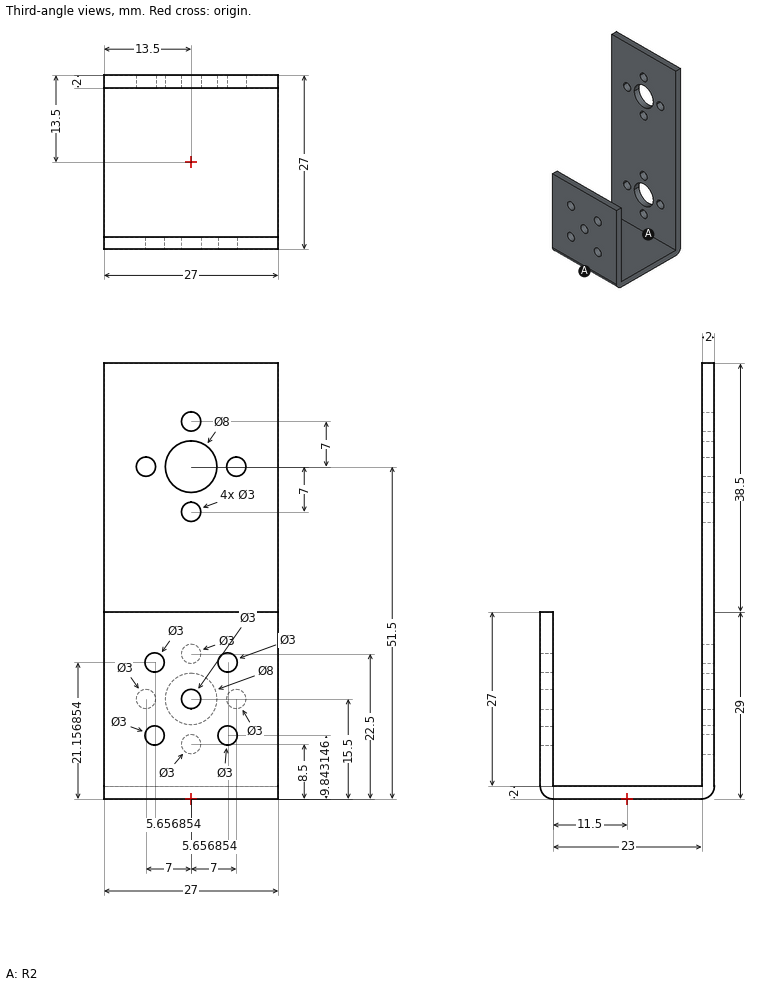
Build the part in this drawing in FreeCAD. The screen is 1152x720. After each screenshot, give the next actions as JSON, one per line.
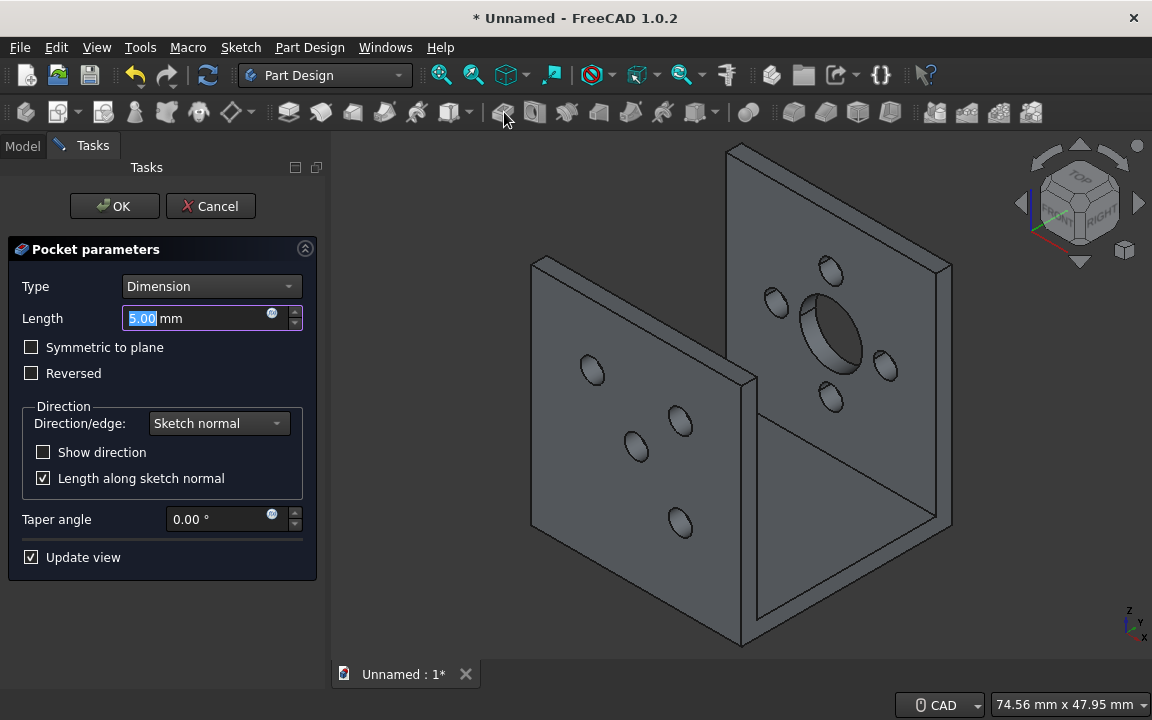
{"action": "left_click", "coordinate": [212, 286]}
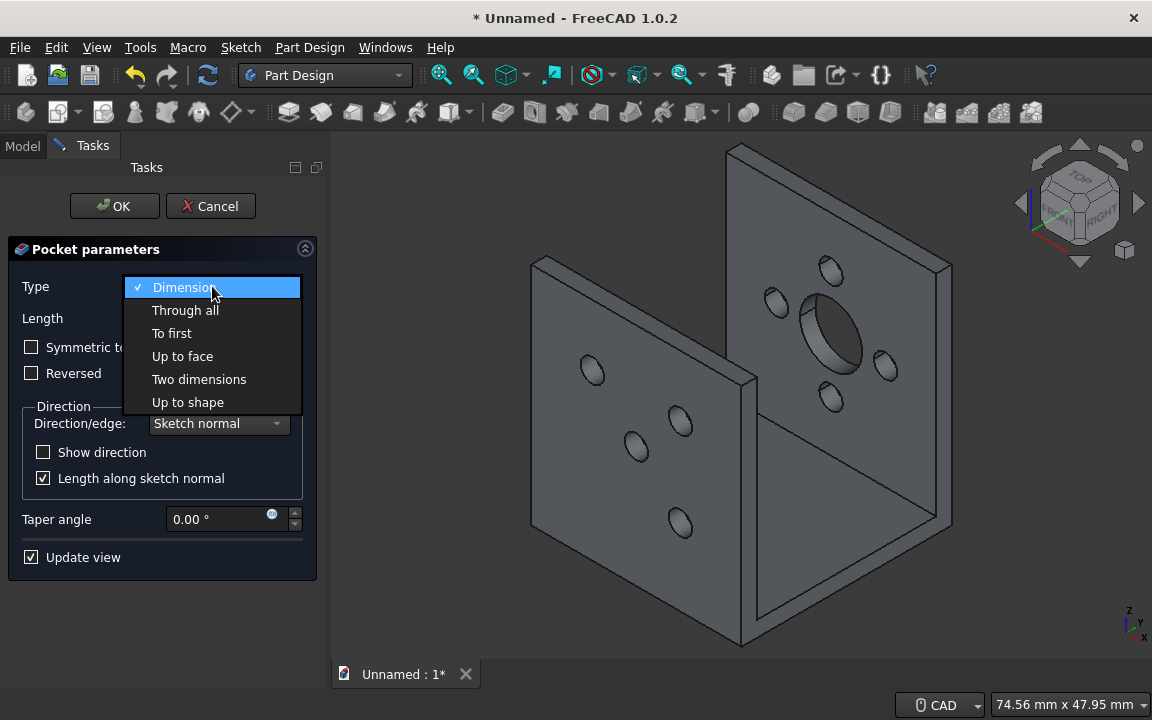
{"action": "left_click", "coordinate": [212, 334]}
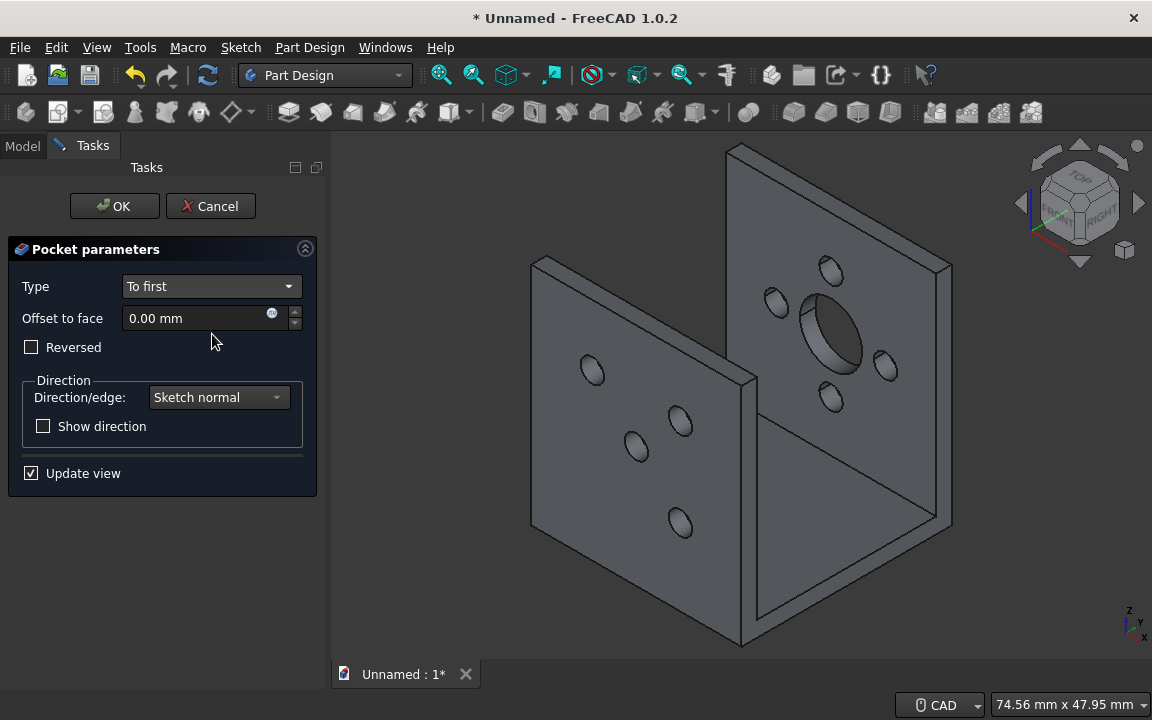
{"action": "left_click", "coordinate": [115, 206]}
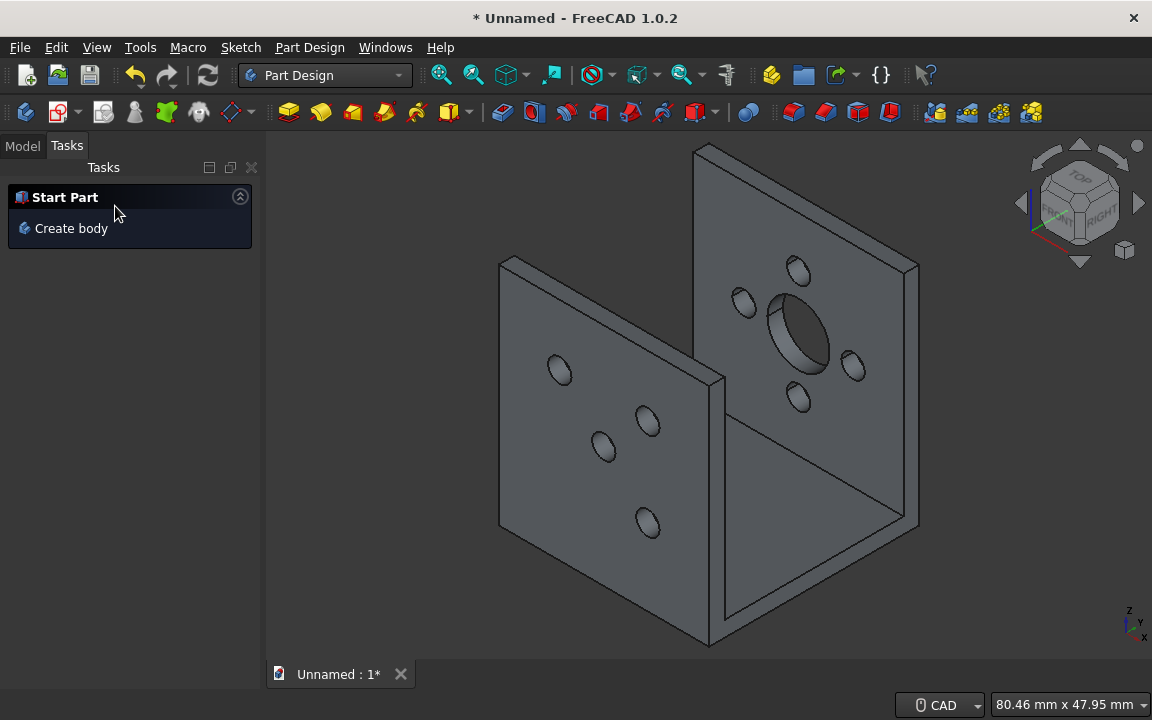
{"action": "left_click", "coordinate": [574, 512]}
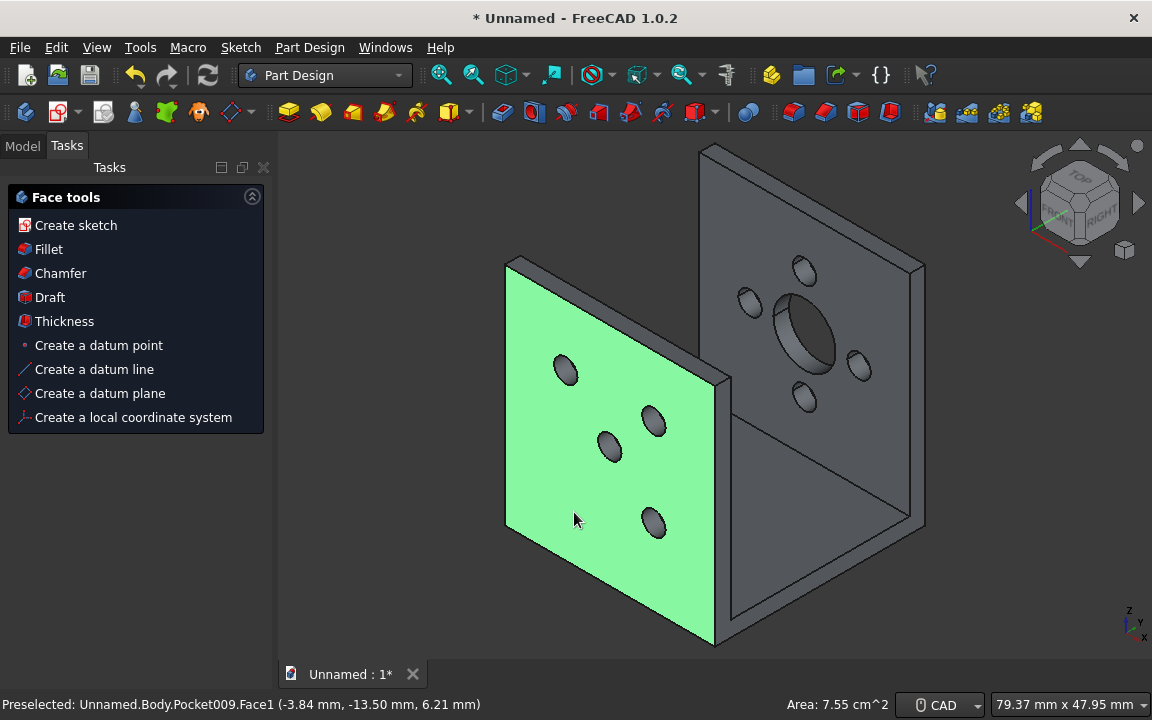
{"action": "left_click", "coordinate": [58, 112]}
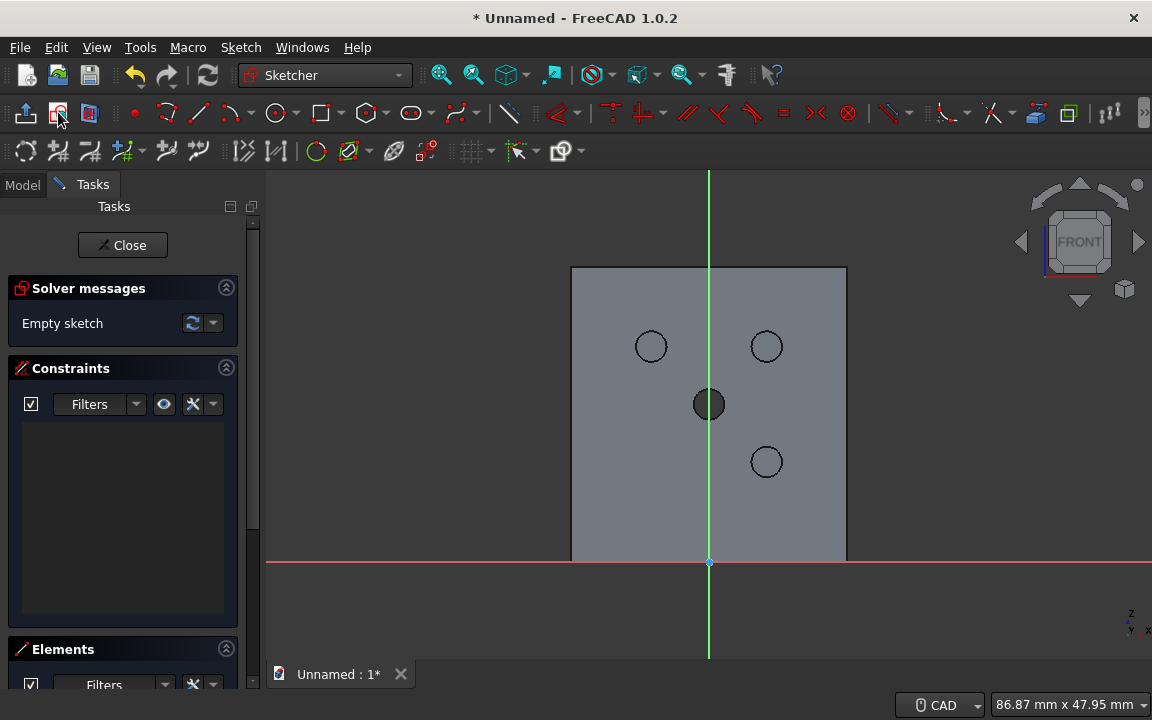
{"action": "scroll", "coordinate": [652, 467], "scroll_direction": "up", "scroll_amount": 12}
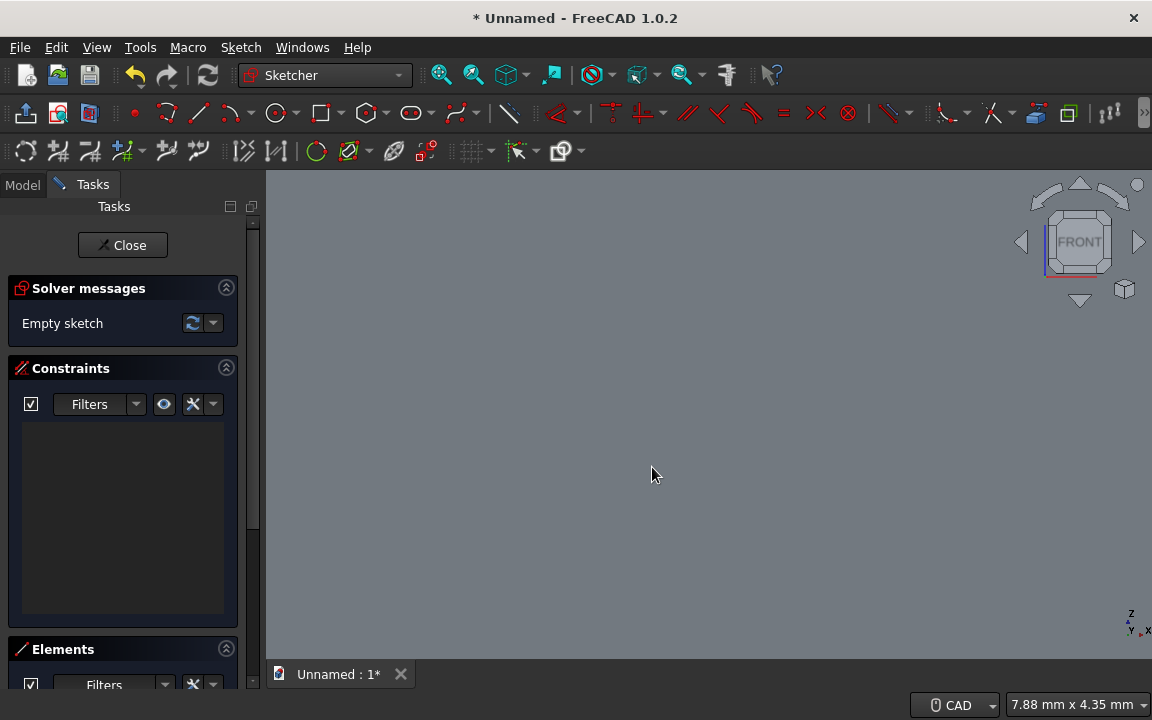
{"action": "key", "text": "g c"}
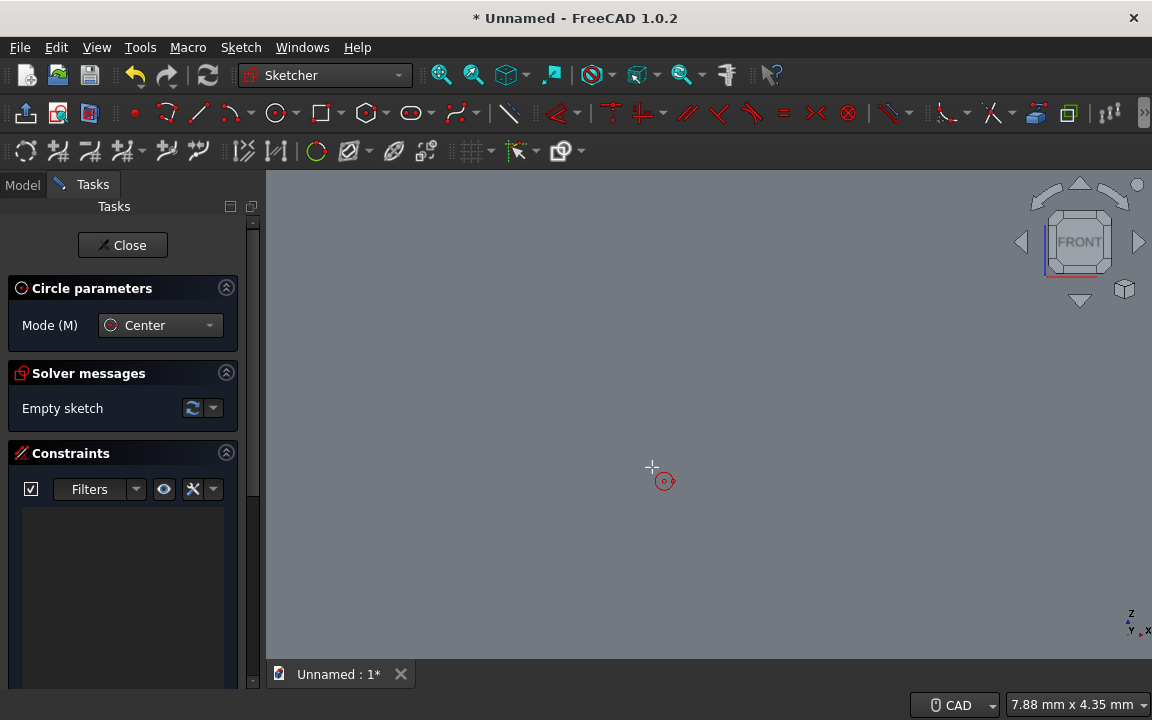
{"action": "left_click", "coordinate": [640, 406]}
{"action": "left_click", "coordinate": [759, 286]}
{"action": "key", "text": "Escape"}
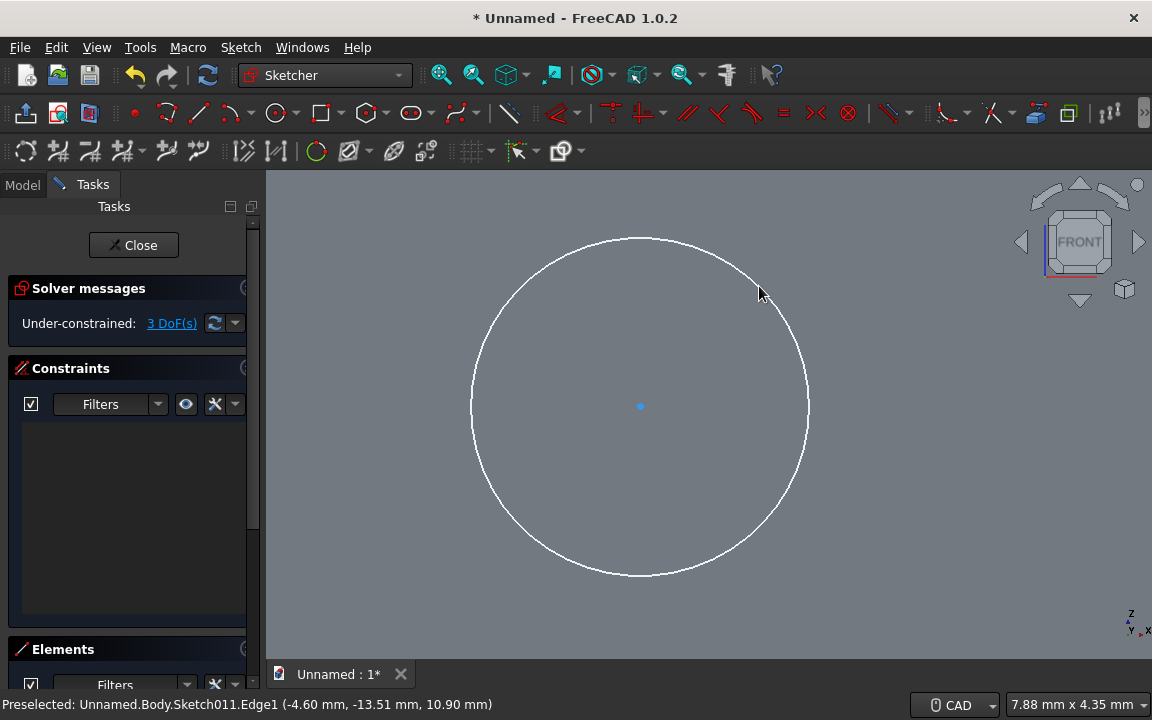
{"action": "key", "text": "d"}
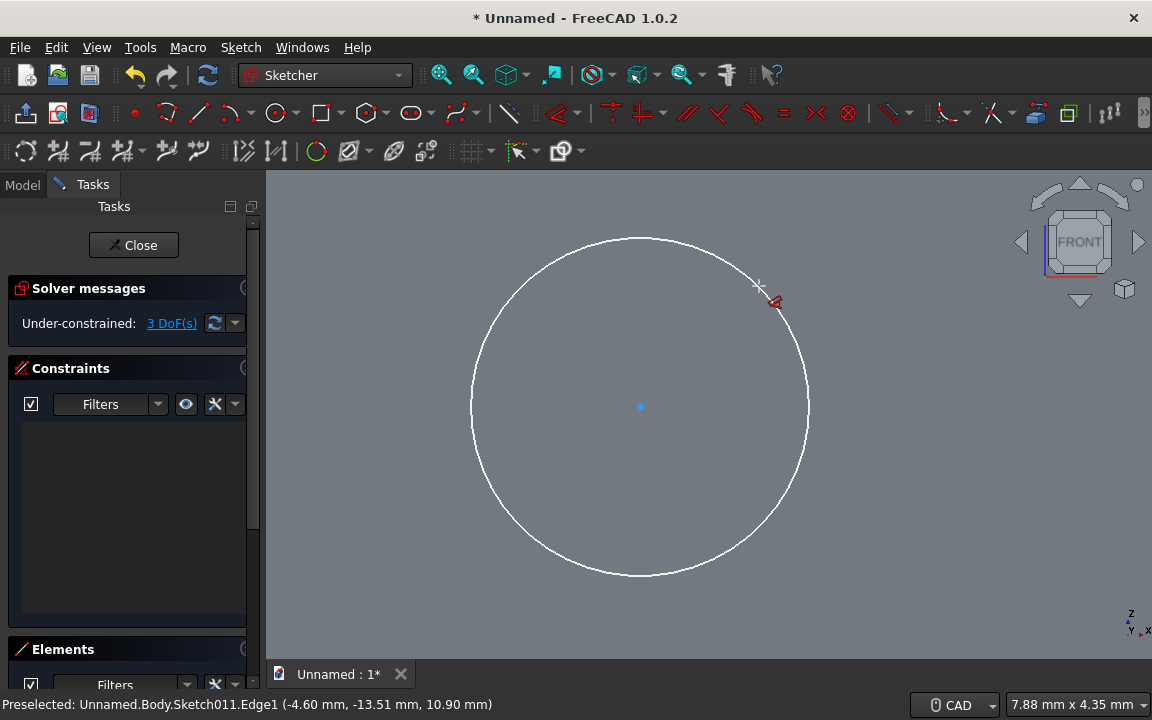
{"action": "left_click", "coordinate": [759, 287]}
{"action": "left_click", "coordinate": [782, 264]}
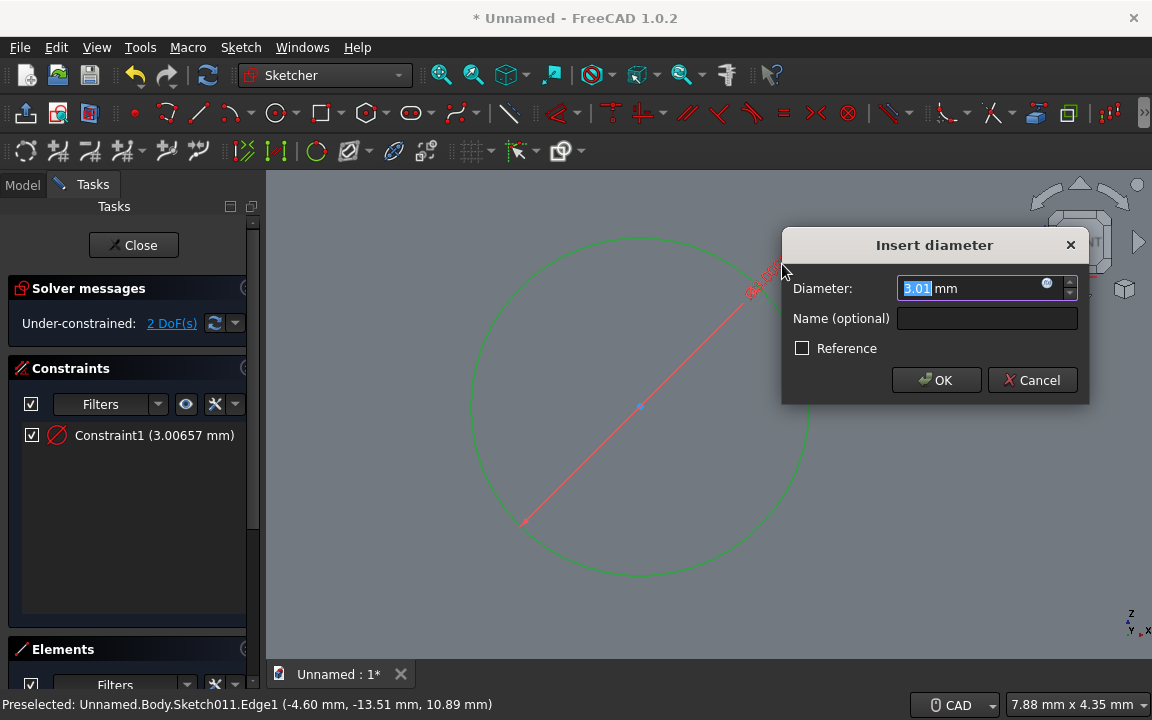
{"action": "type", "text": "3"}
{"action": "key", "text": "Return"}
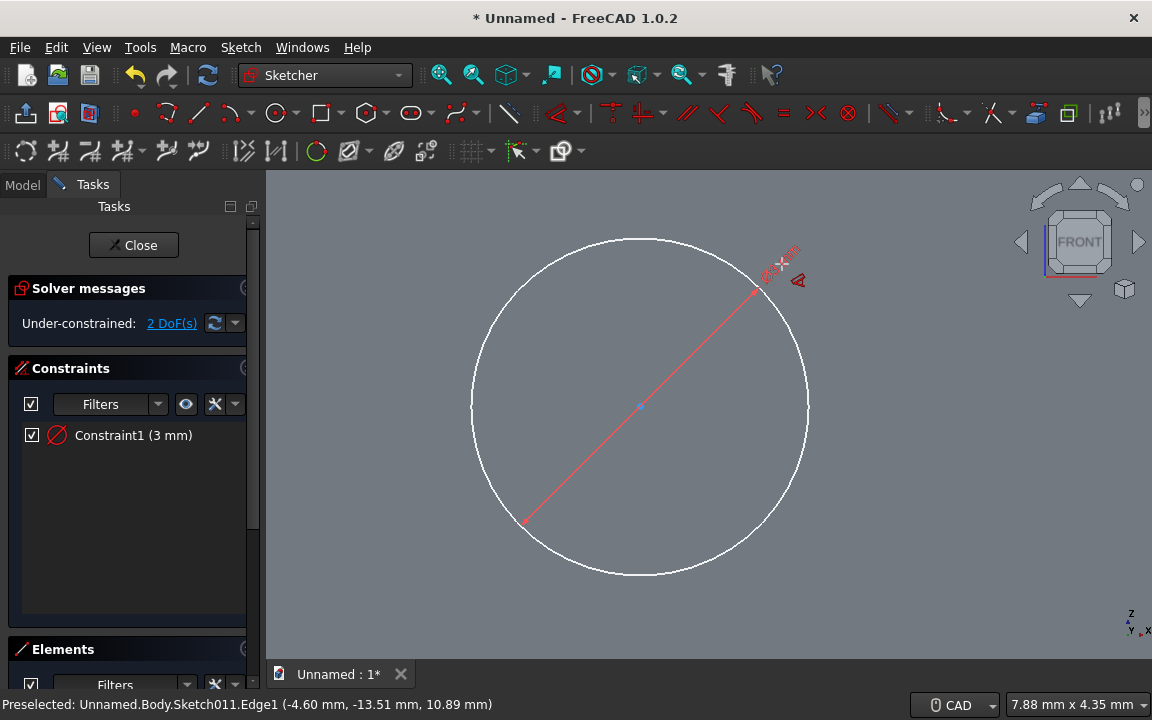
{"action": "left_click", "coordinate": [640, 407]}
{"action": "left_click", "coordinate": [734, 373]}